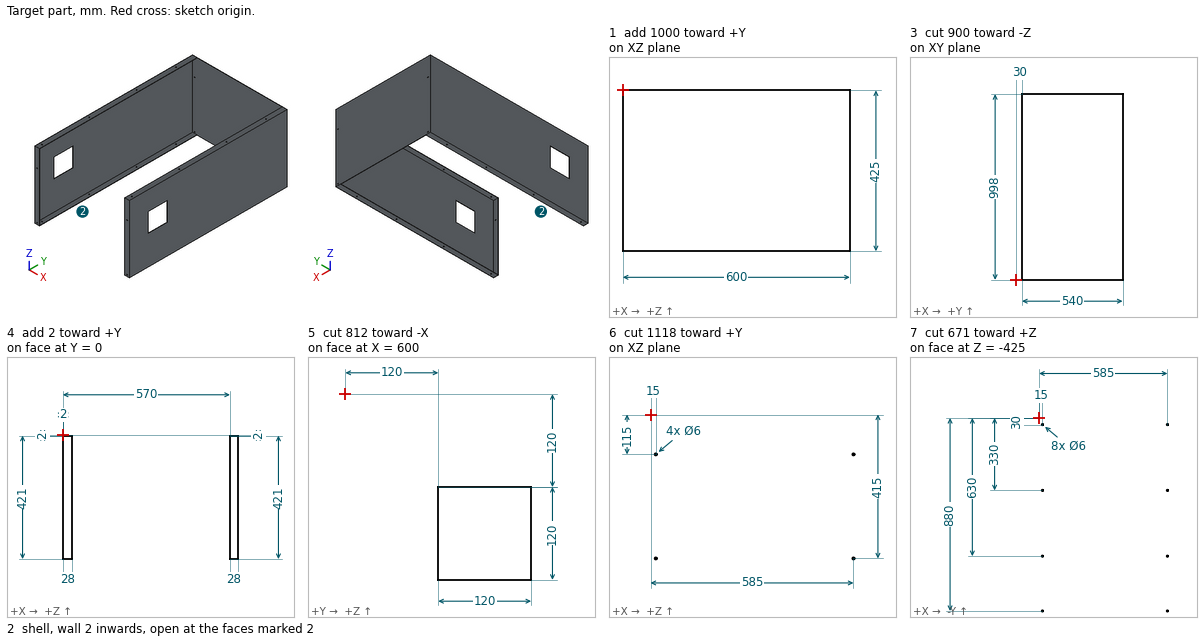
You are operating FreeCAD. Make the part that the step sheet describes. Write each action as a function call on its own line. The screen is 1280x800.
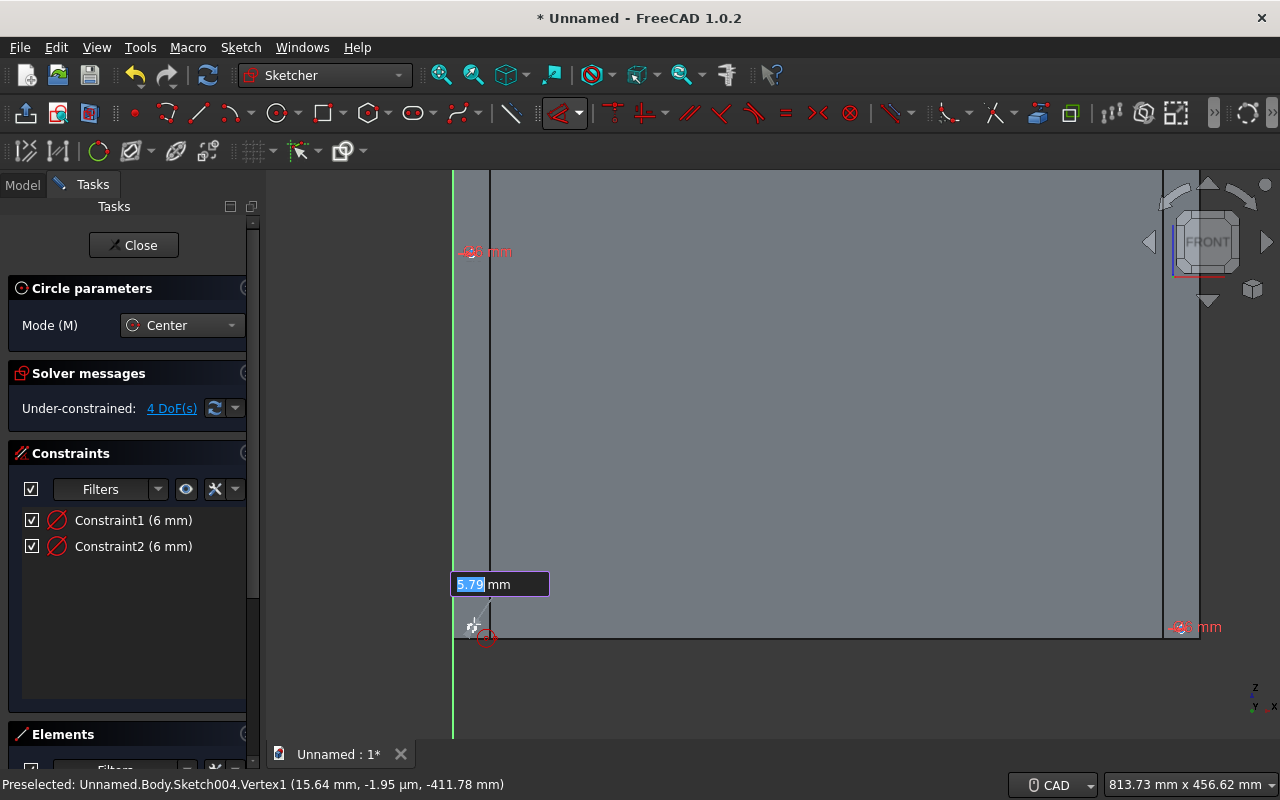
text(6)
key(Return)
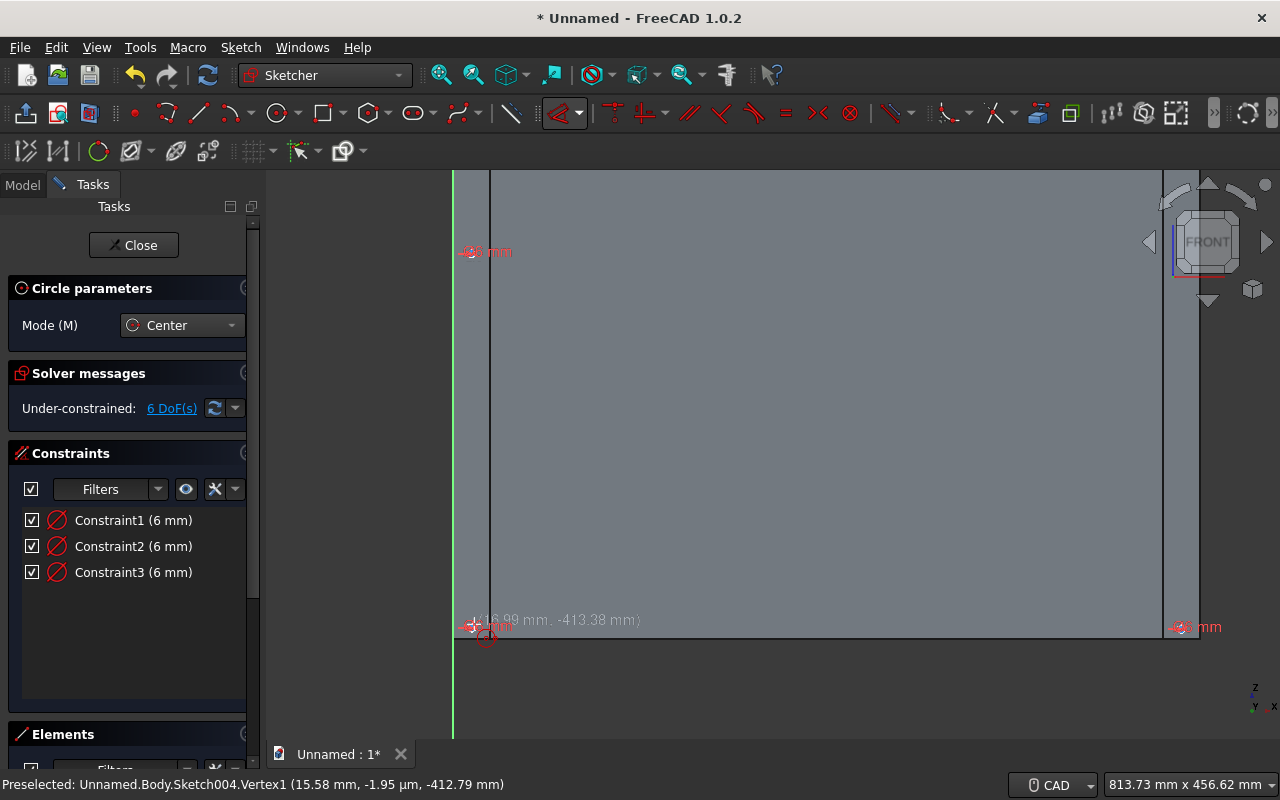
scroll(471, 626, down, 2)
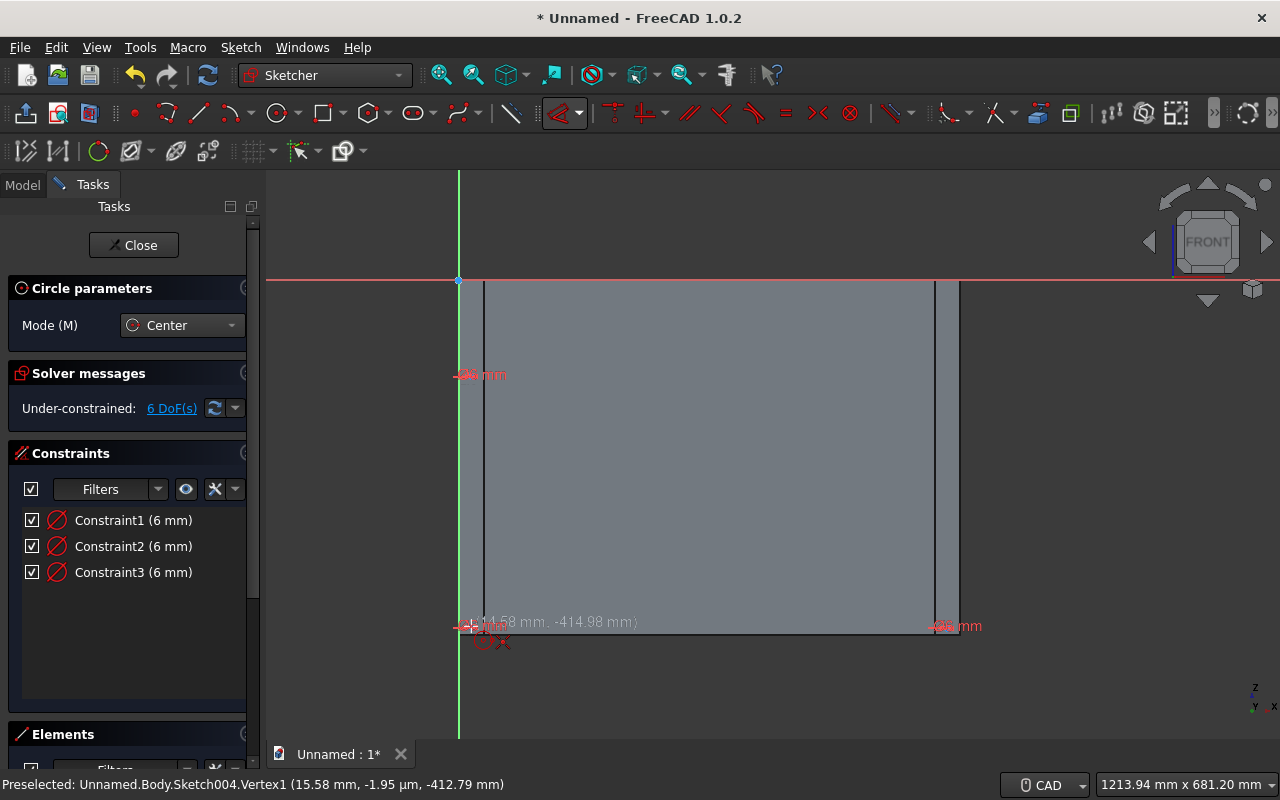
scroll(948, 376, up, 12)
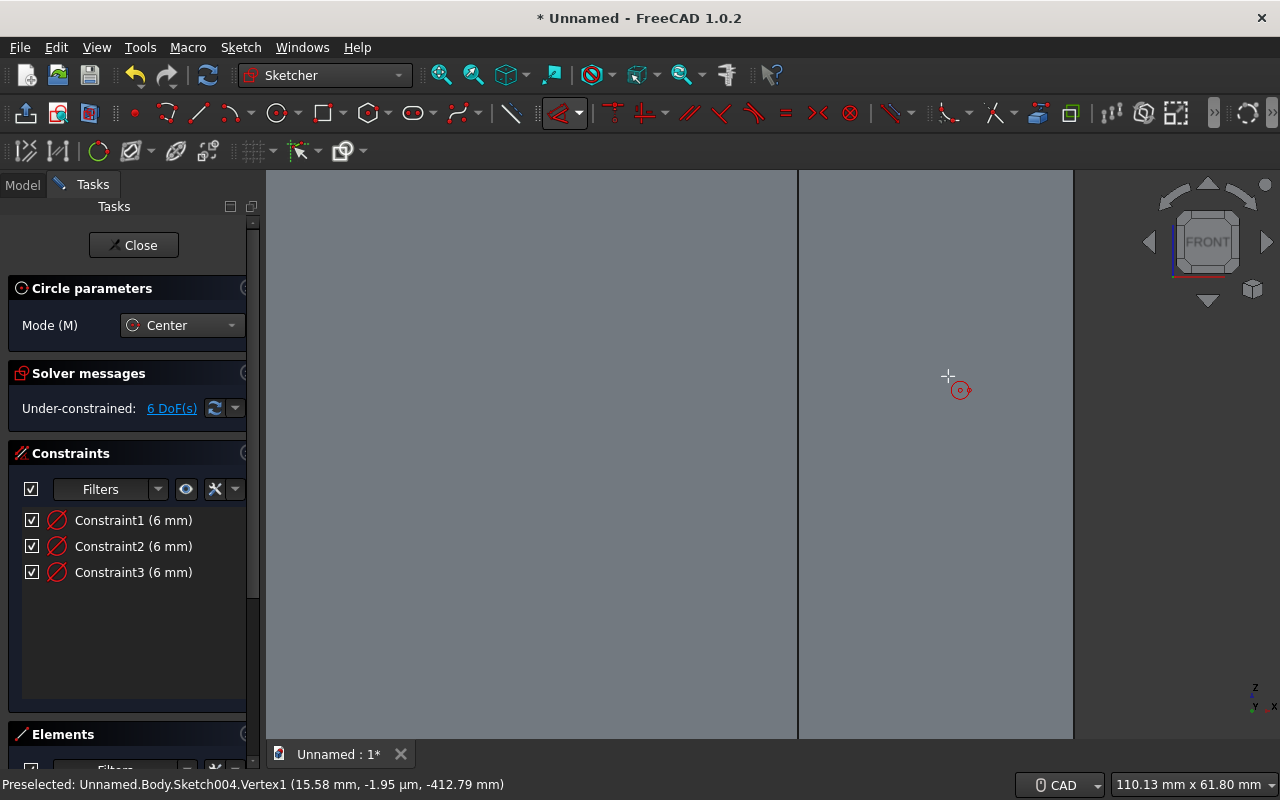
scroll(949, 376, down, 12)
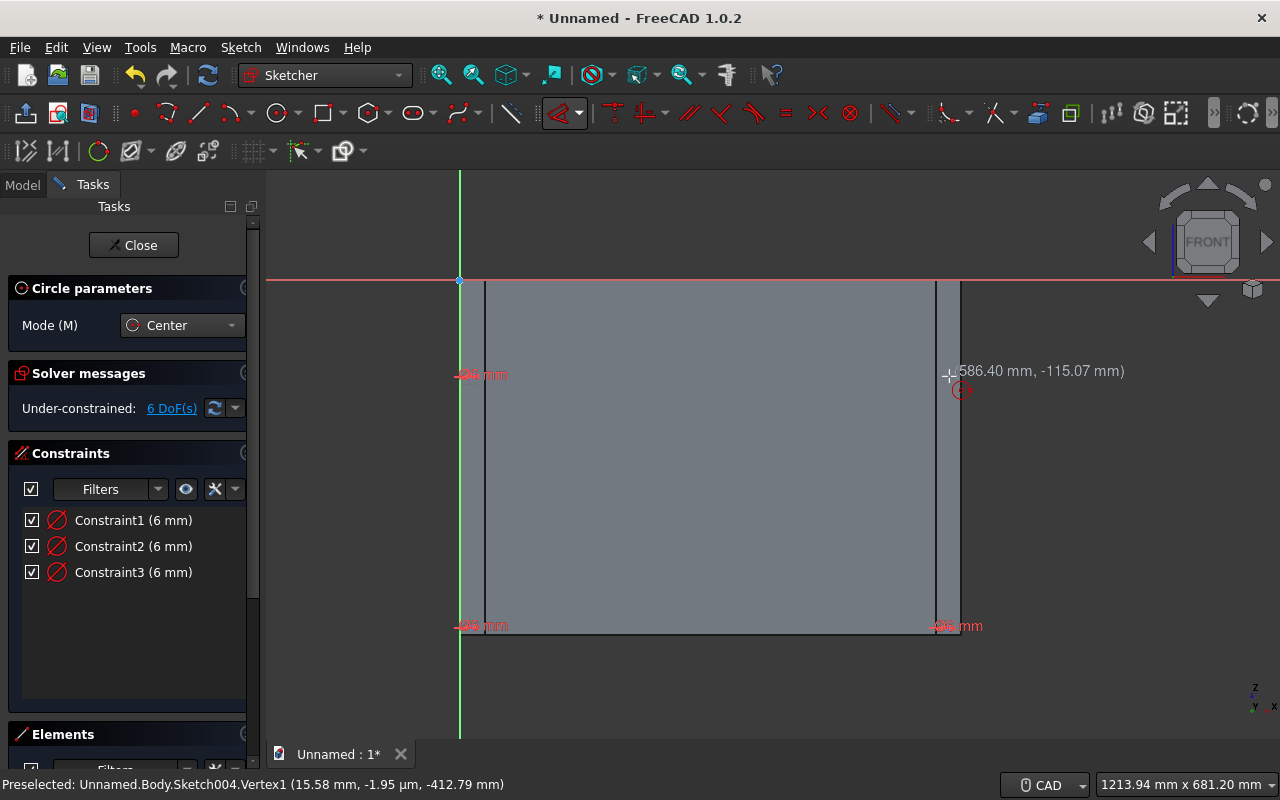
click(948, 376)
move(950, 375)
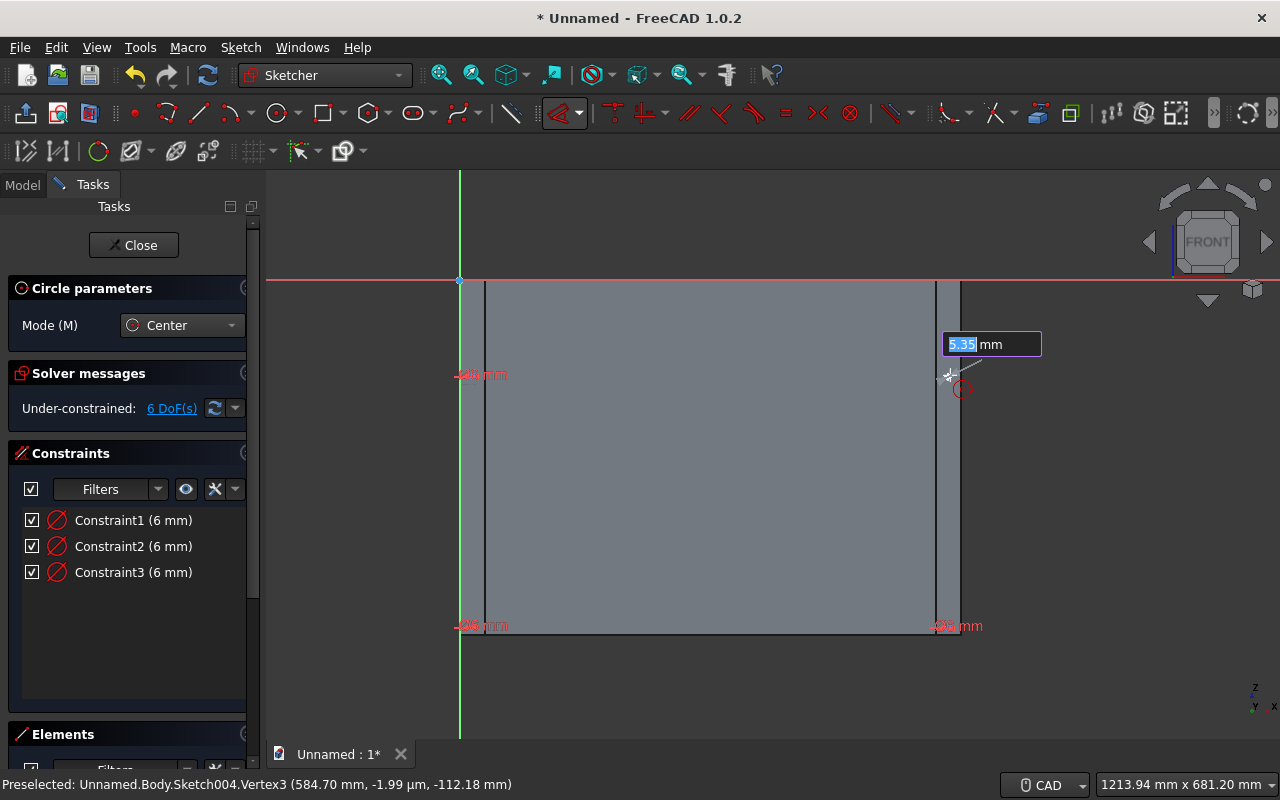
text(6)
key(Return)
key(Escape)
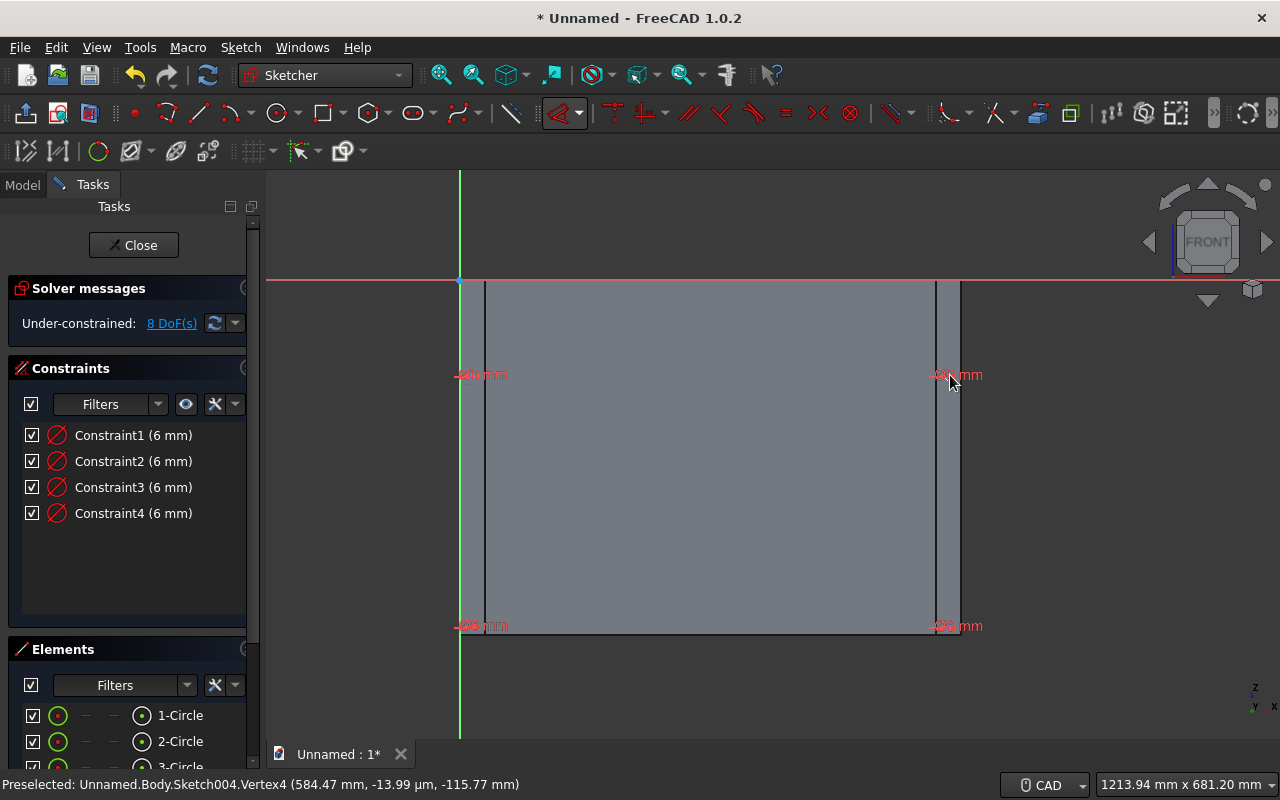
click(472, 377)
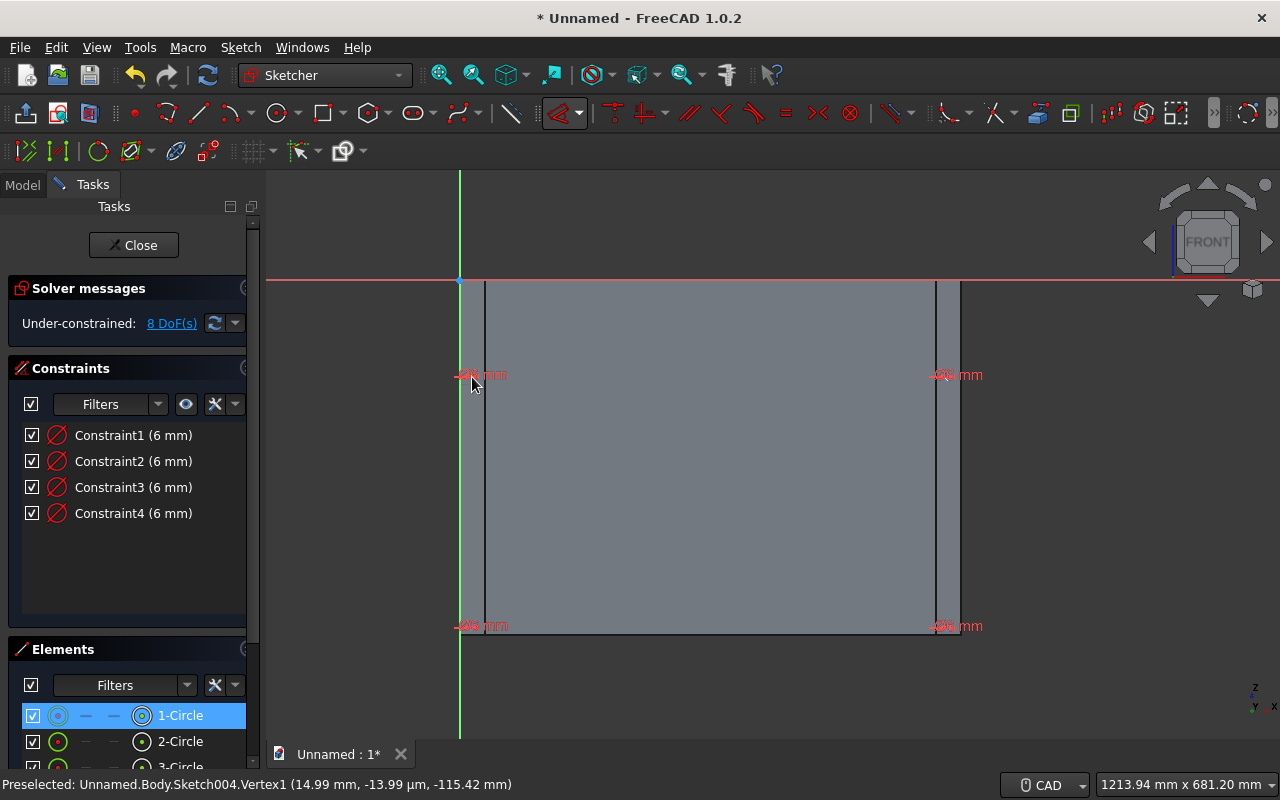
click(473, 628)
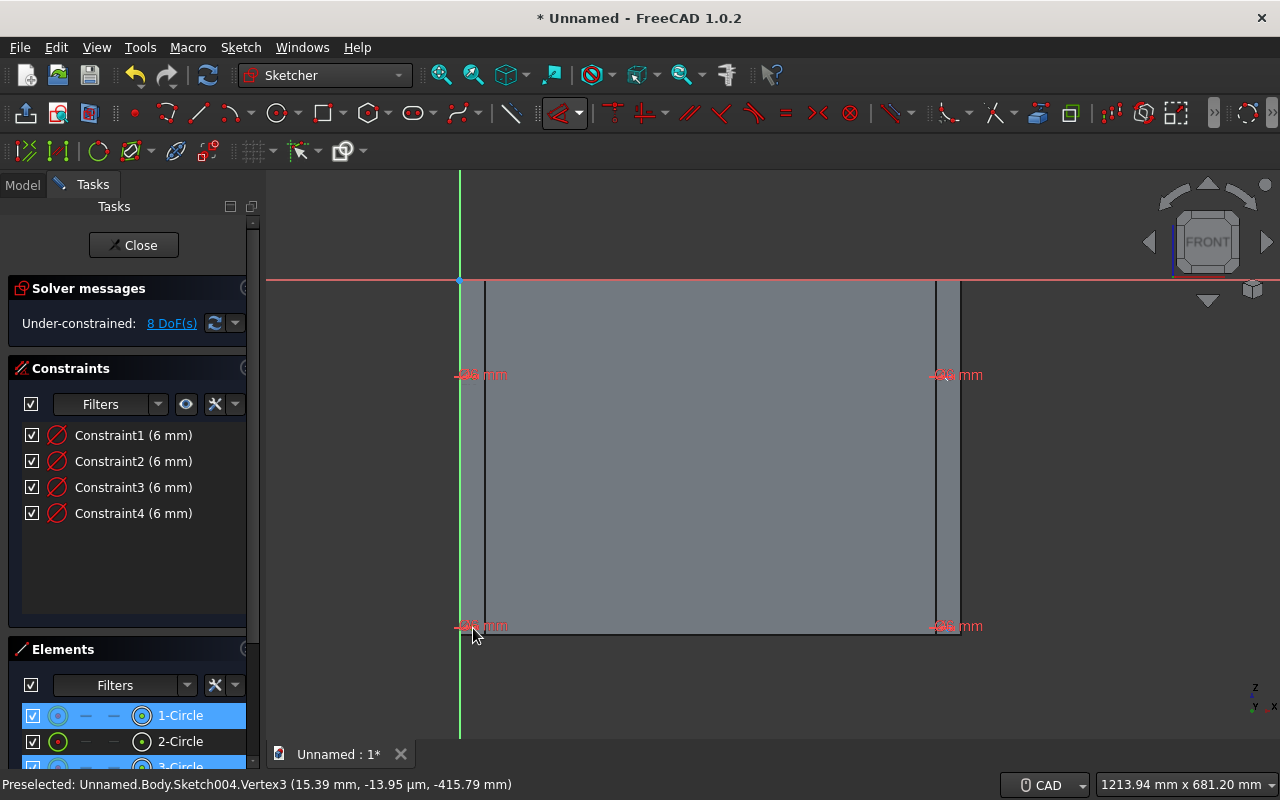
click(668, 114)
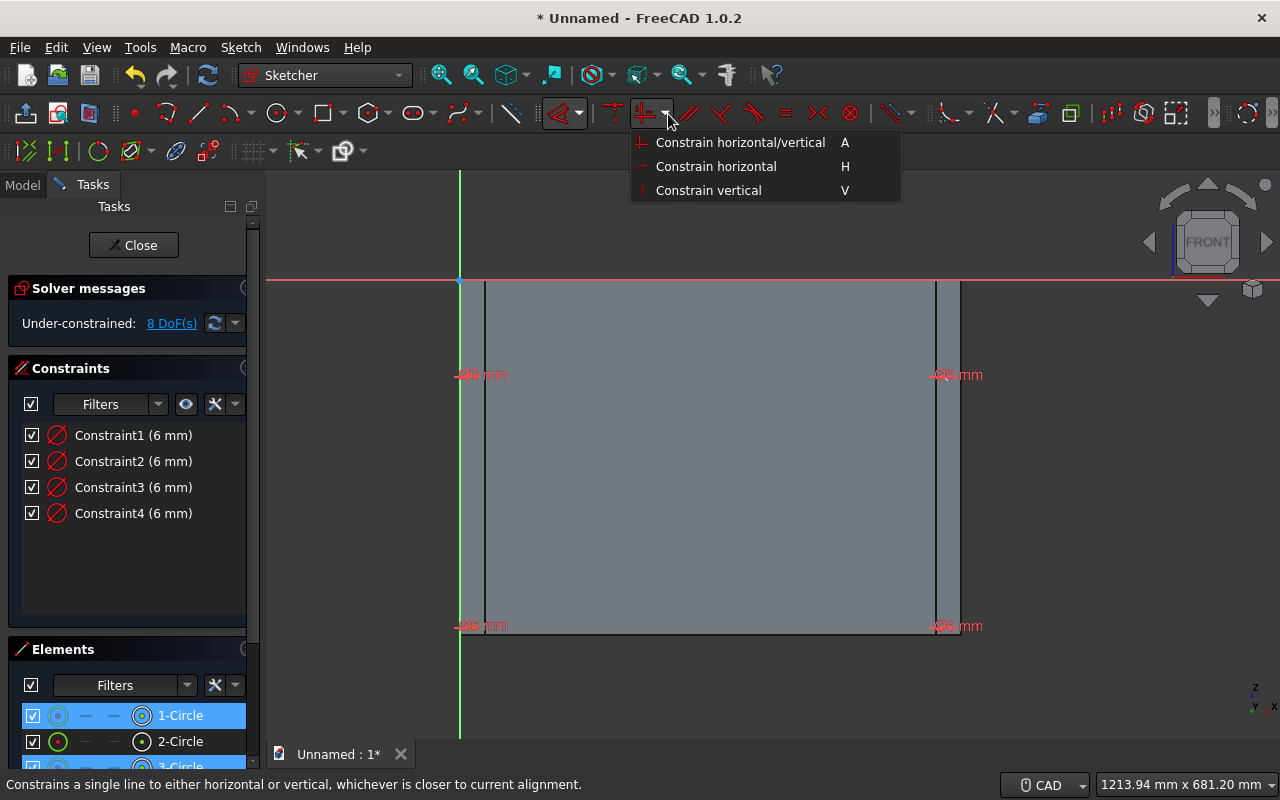
click(766, 190)